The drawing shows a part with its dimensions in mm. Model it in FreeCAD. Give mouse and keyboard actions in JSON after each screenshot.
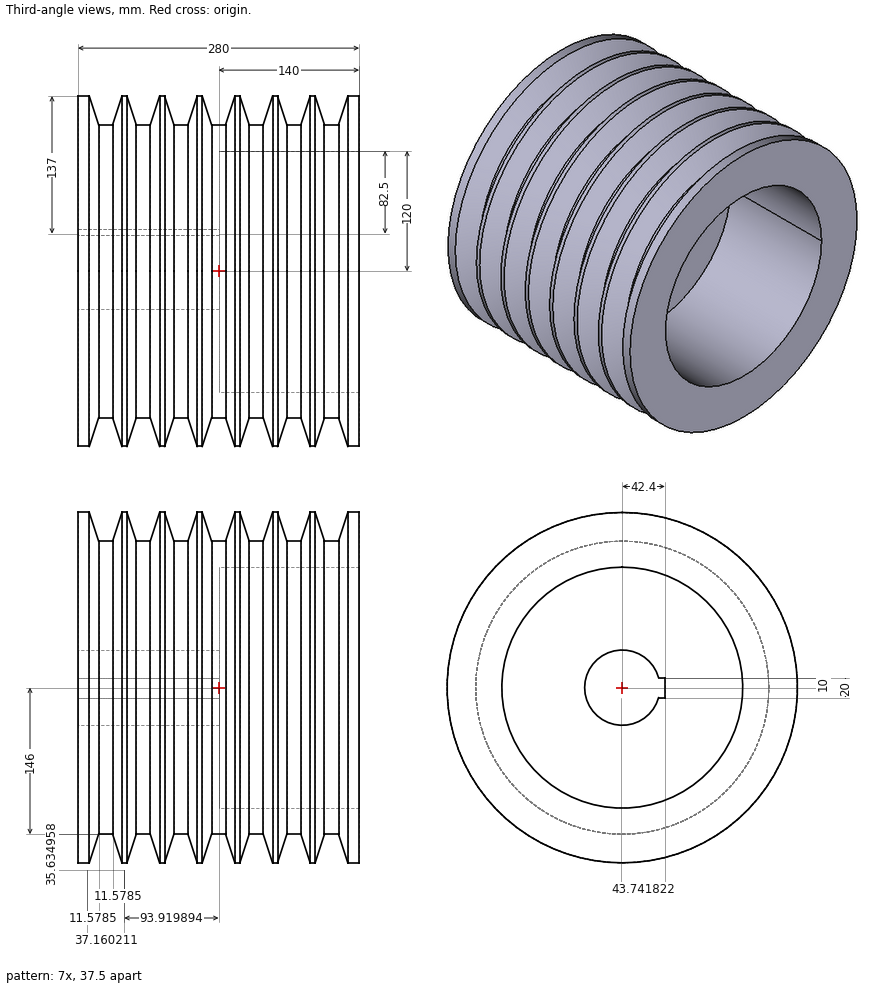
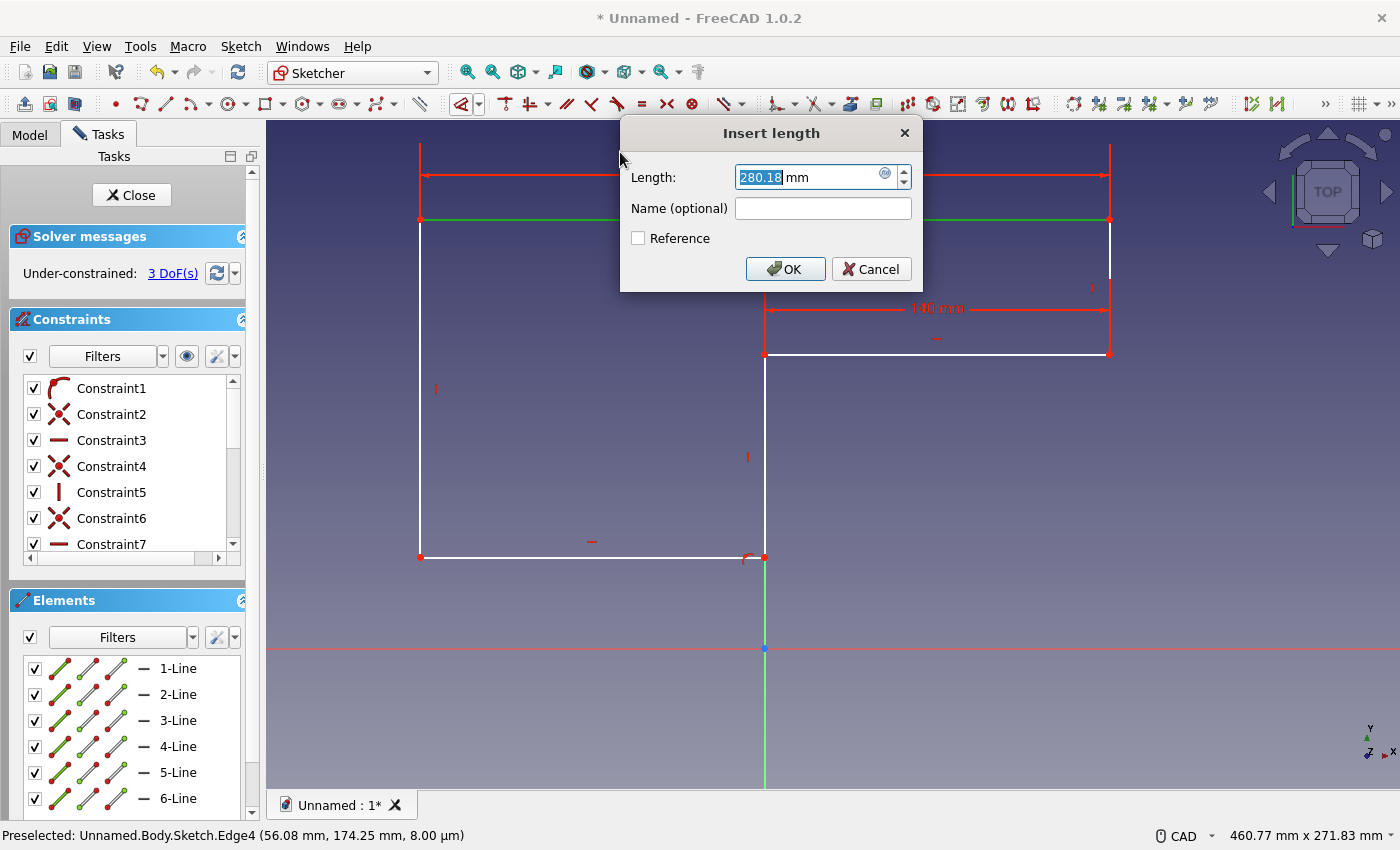
{"action": "type", "text": "280"}
{"action": "key", "text": "Return"}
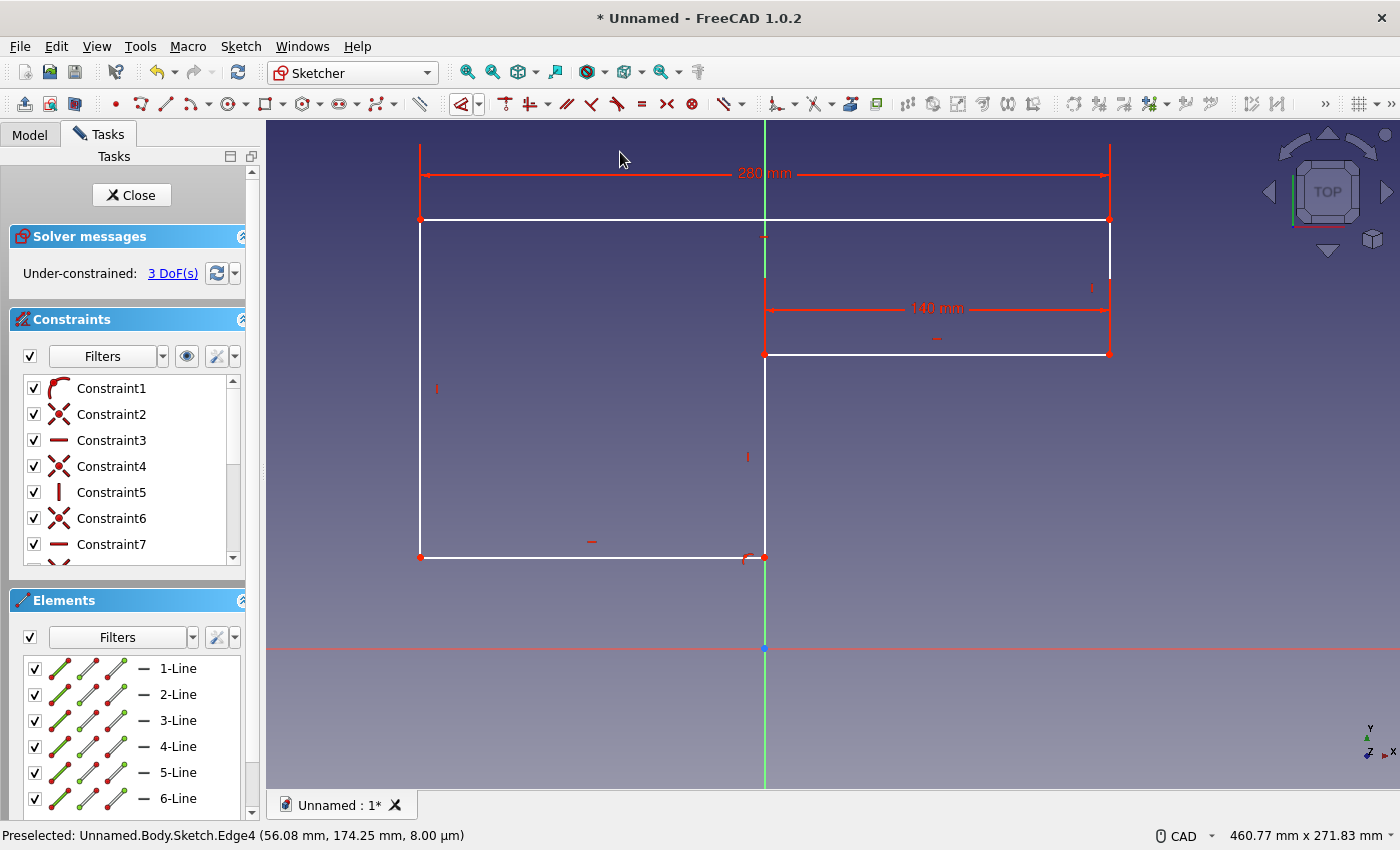
{"action": "left_click", "coordinate": [420, 321]}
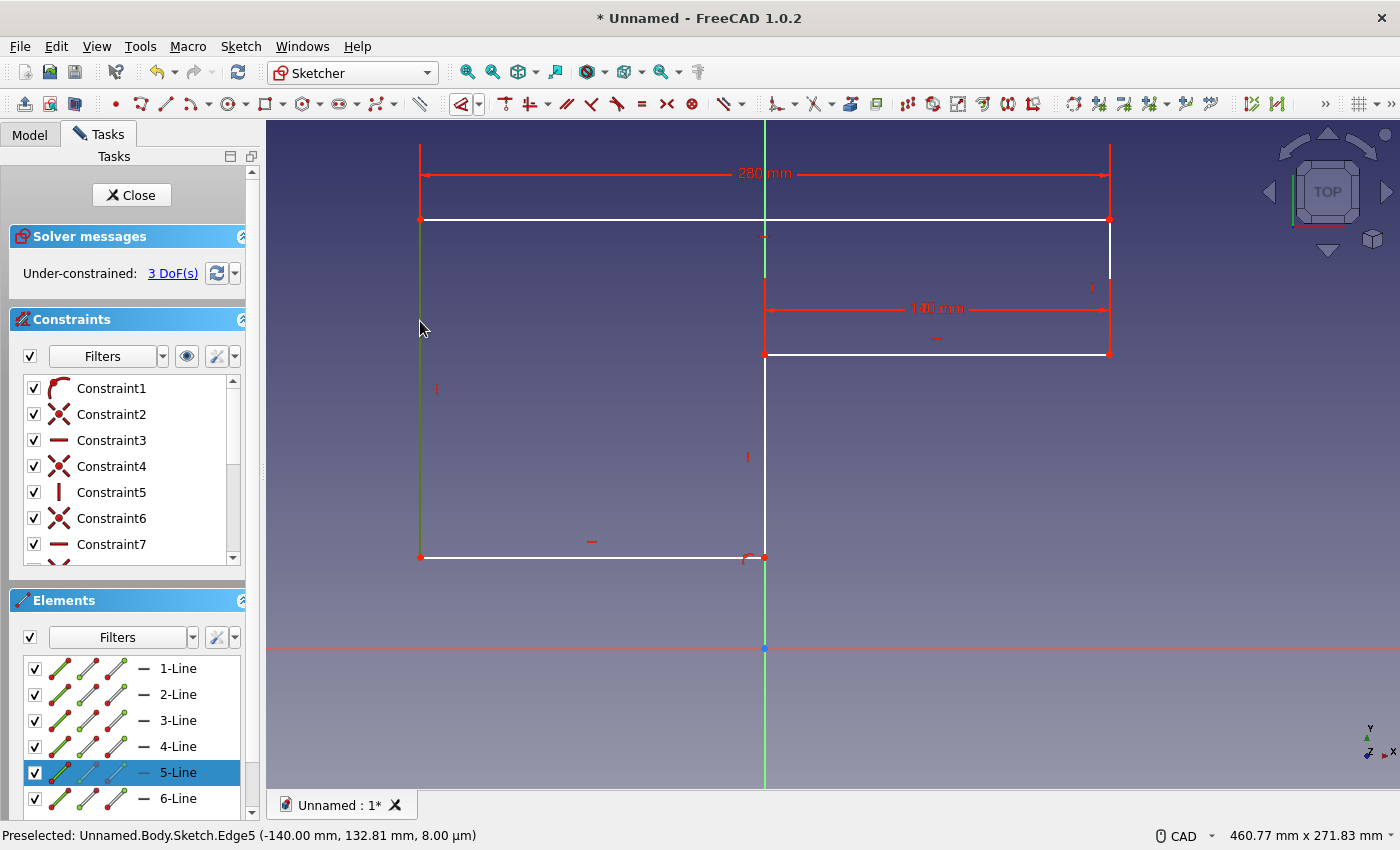
{"action": "left_click", "coordinate": [478, 104]}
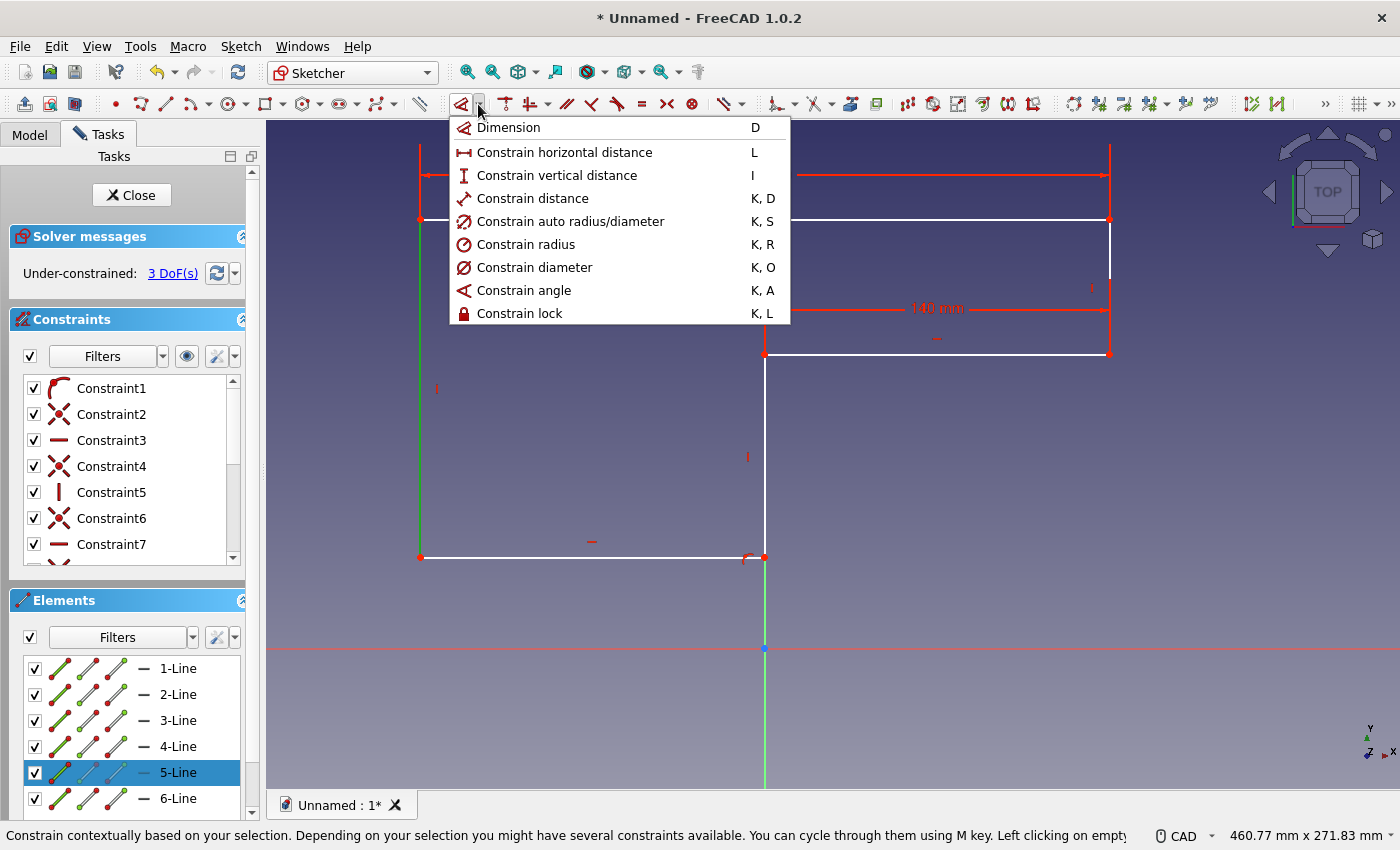
{"action": "left_click", "coordinate": [620, 176]}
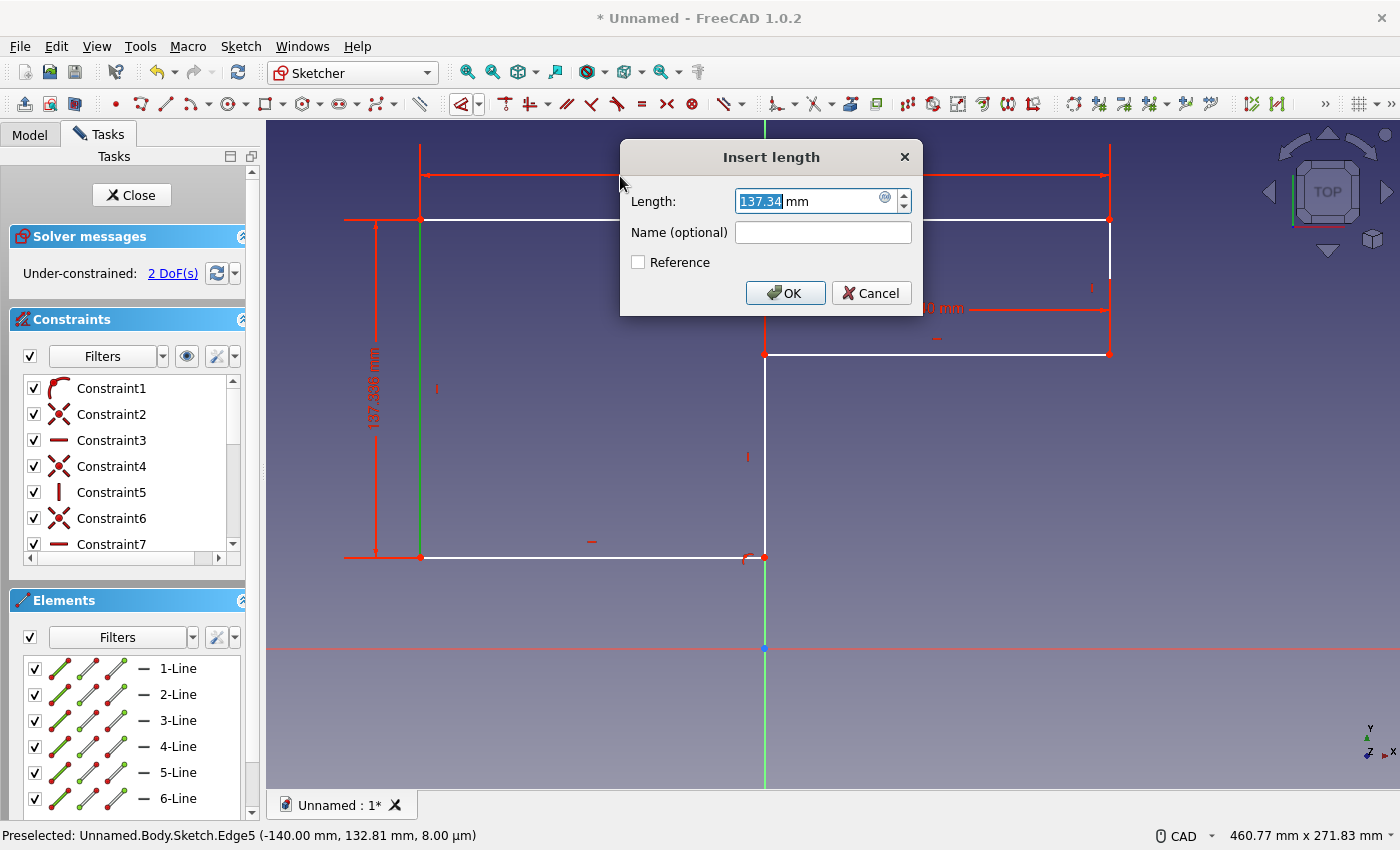
{"action": "type", "text": "137"}
{"action": "key", "text": "Return"}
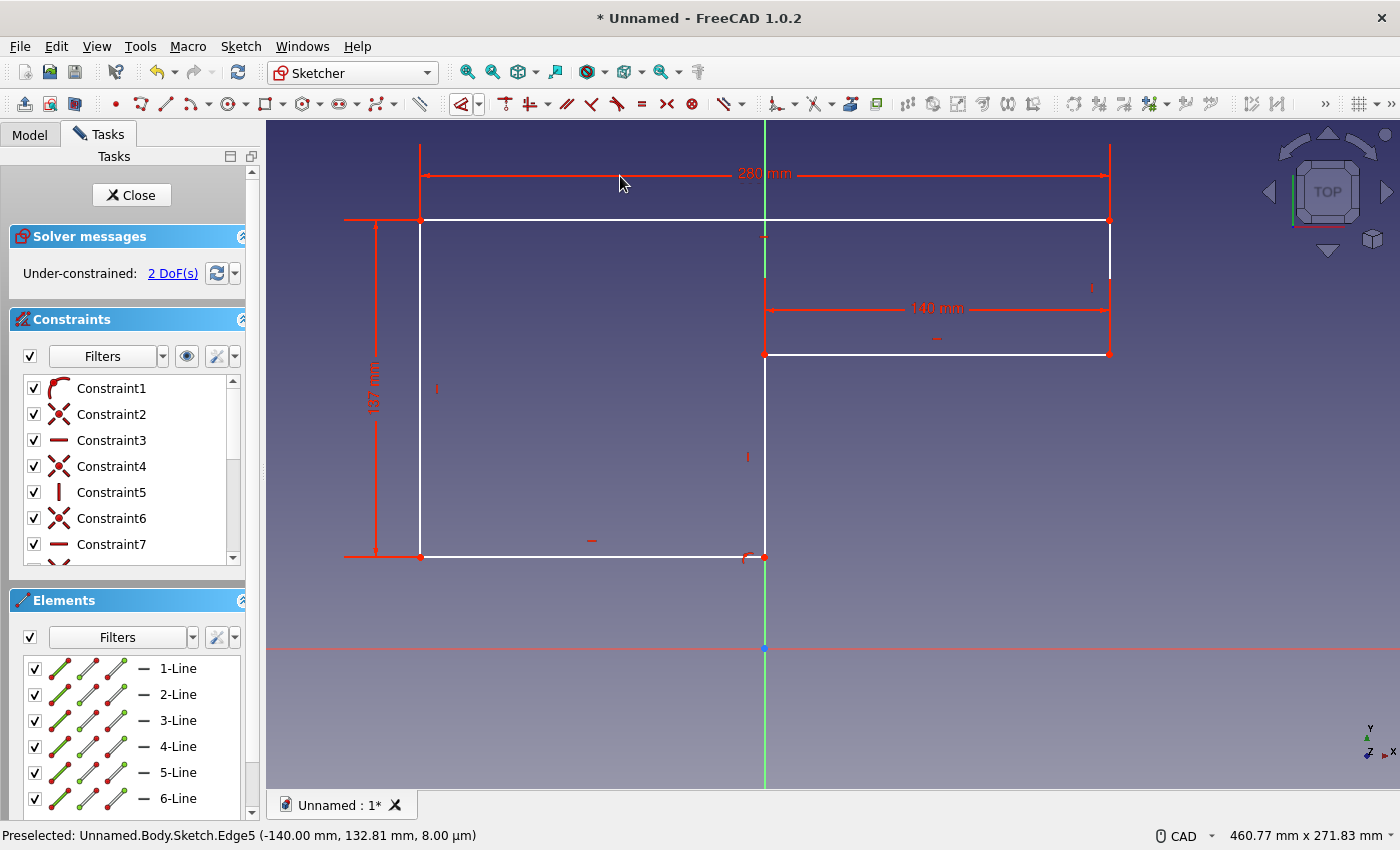
{"action": "left_click", "coordinate": [765, 497]}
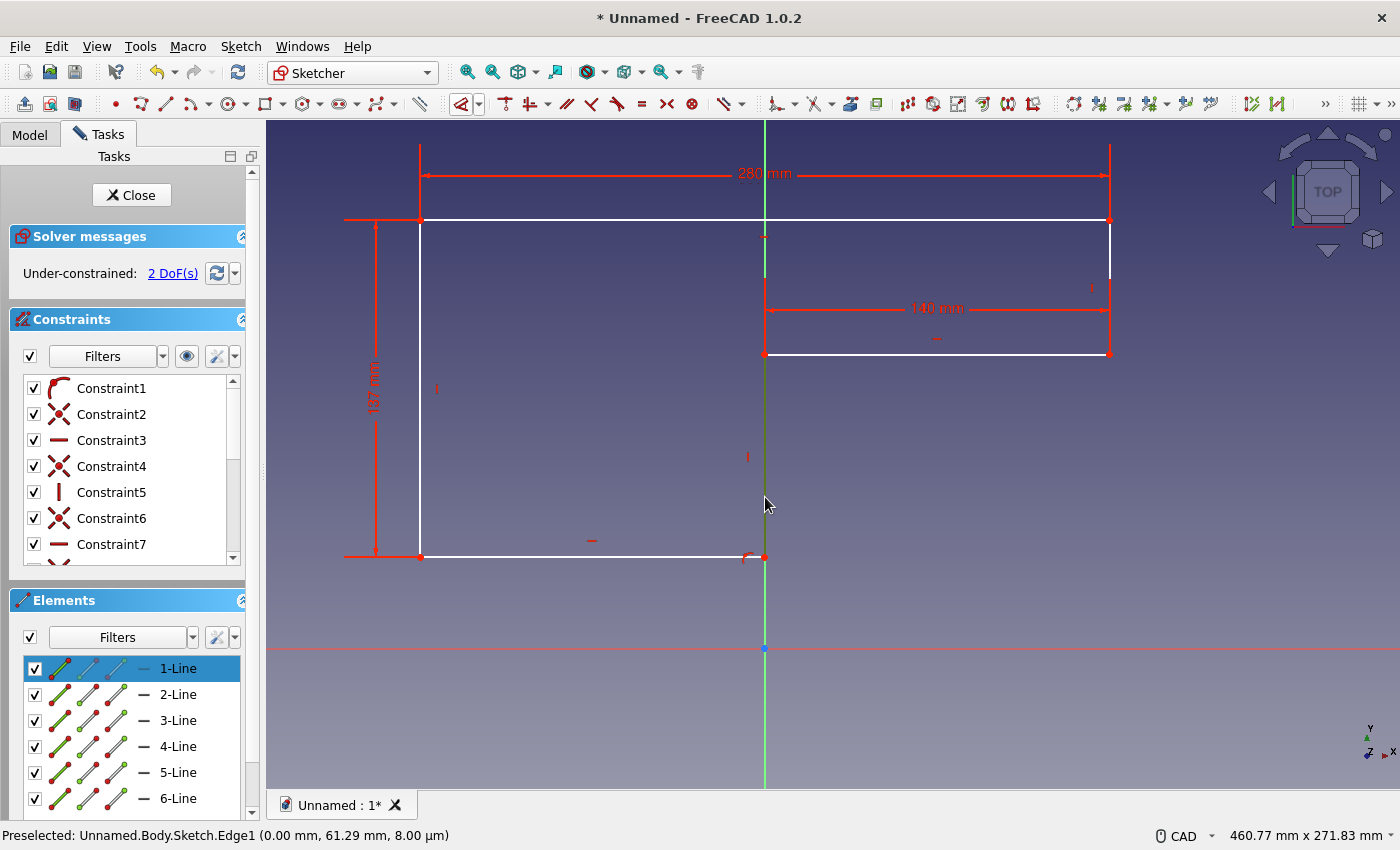
{"action": "key", "text": "i"}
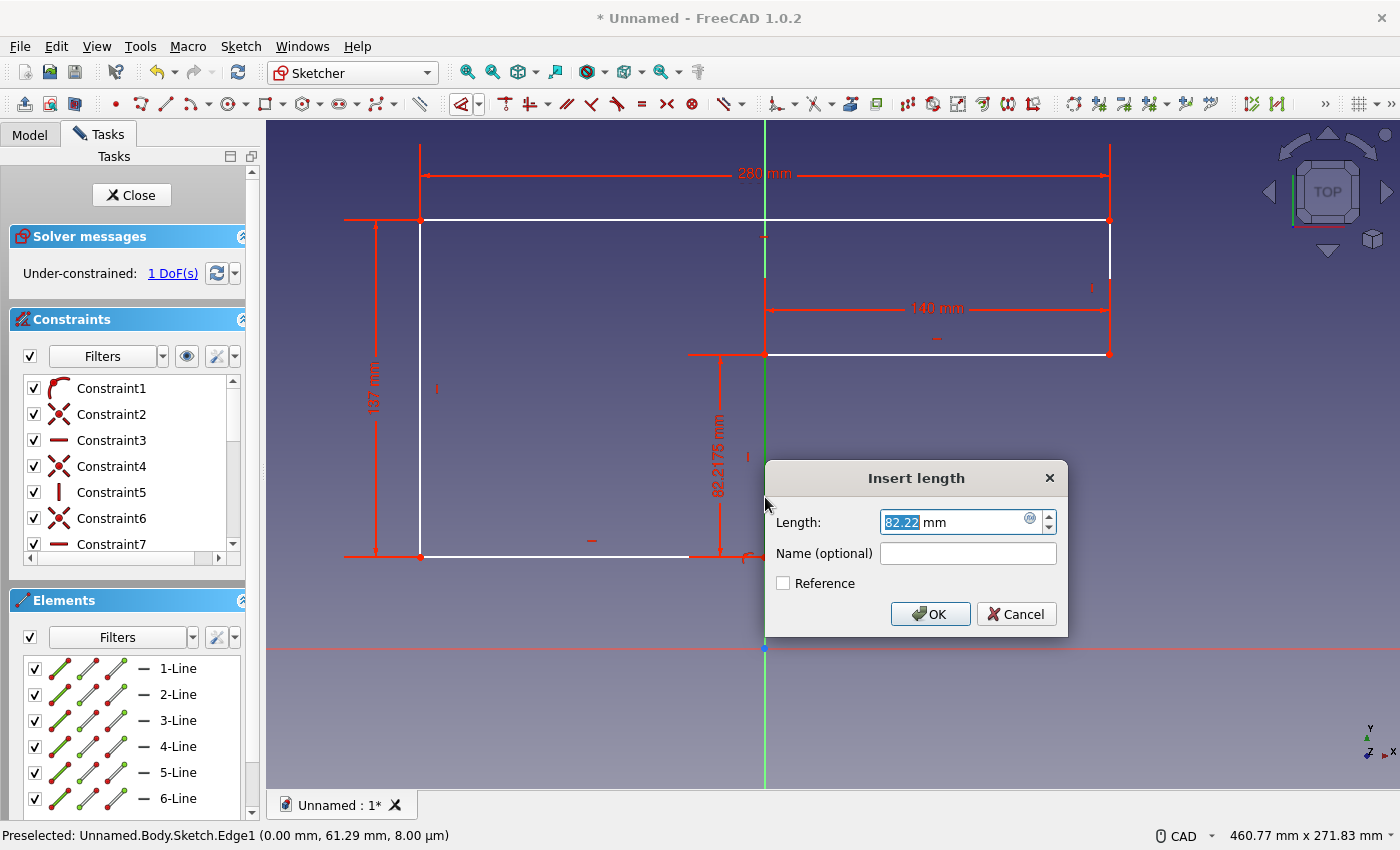
{"action": "type", "text": "82.5"}
{"action": "key", "text": "Return"}